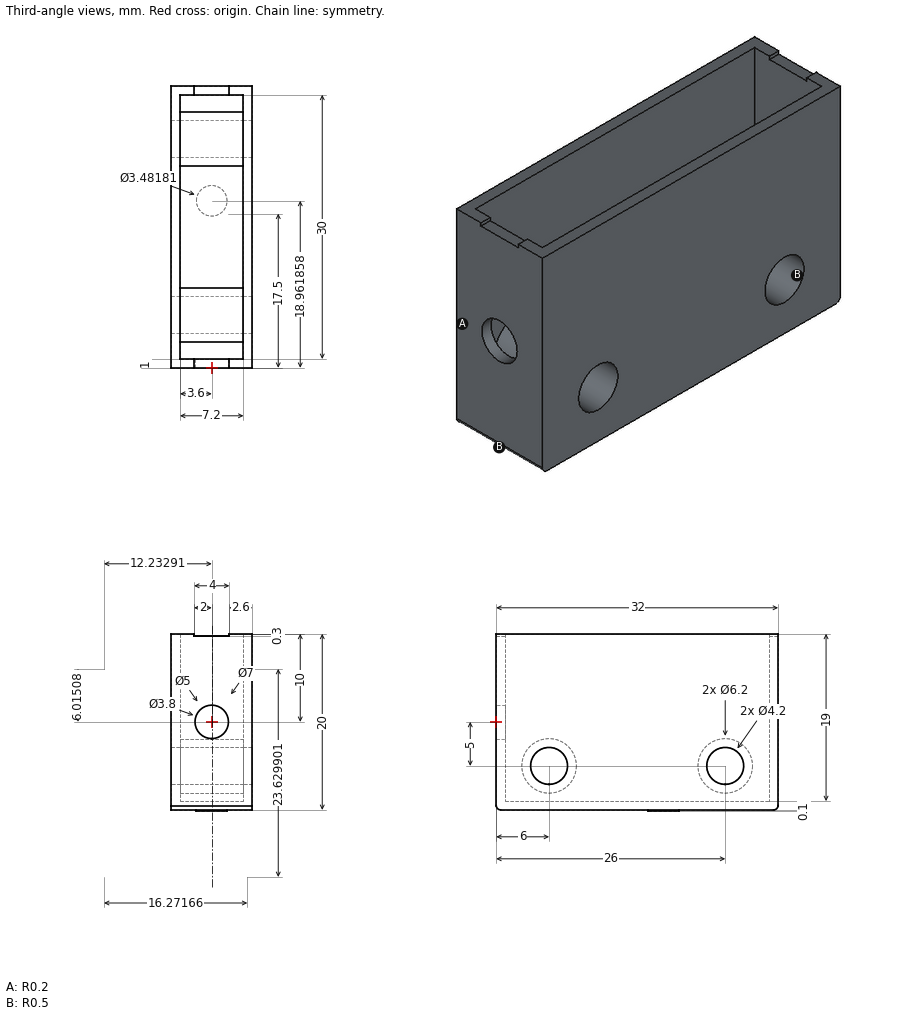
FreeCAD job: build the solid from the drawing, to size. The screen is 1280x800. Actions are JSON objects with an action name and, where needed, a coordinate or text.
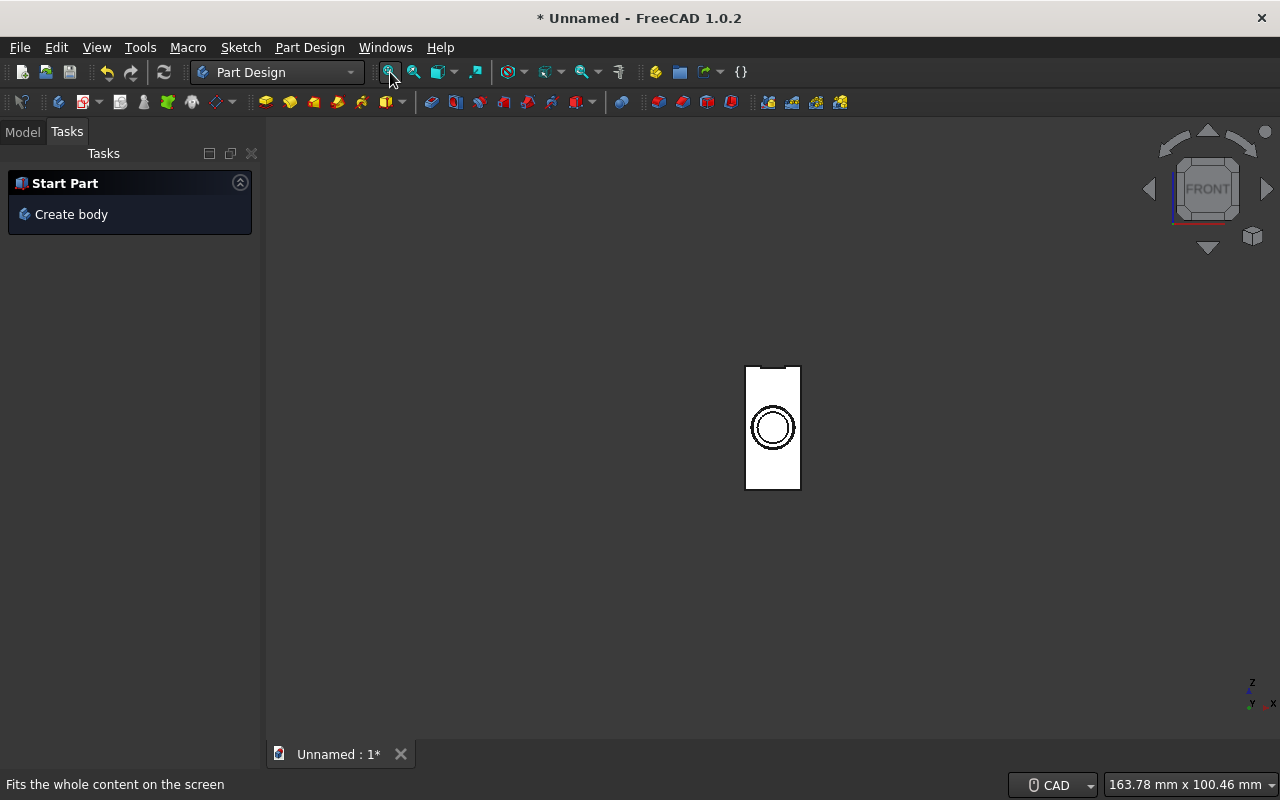
{"action": "key", "text": "3"}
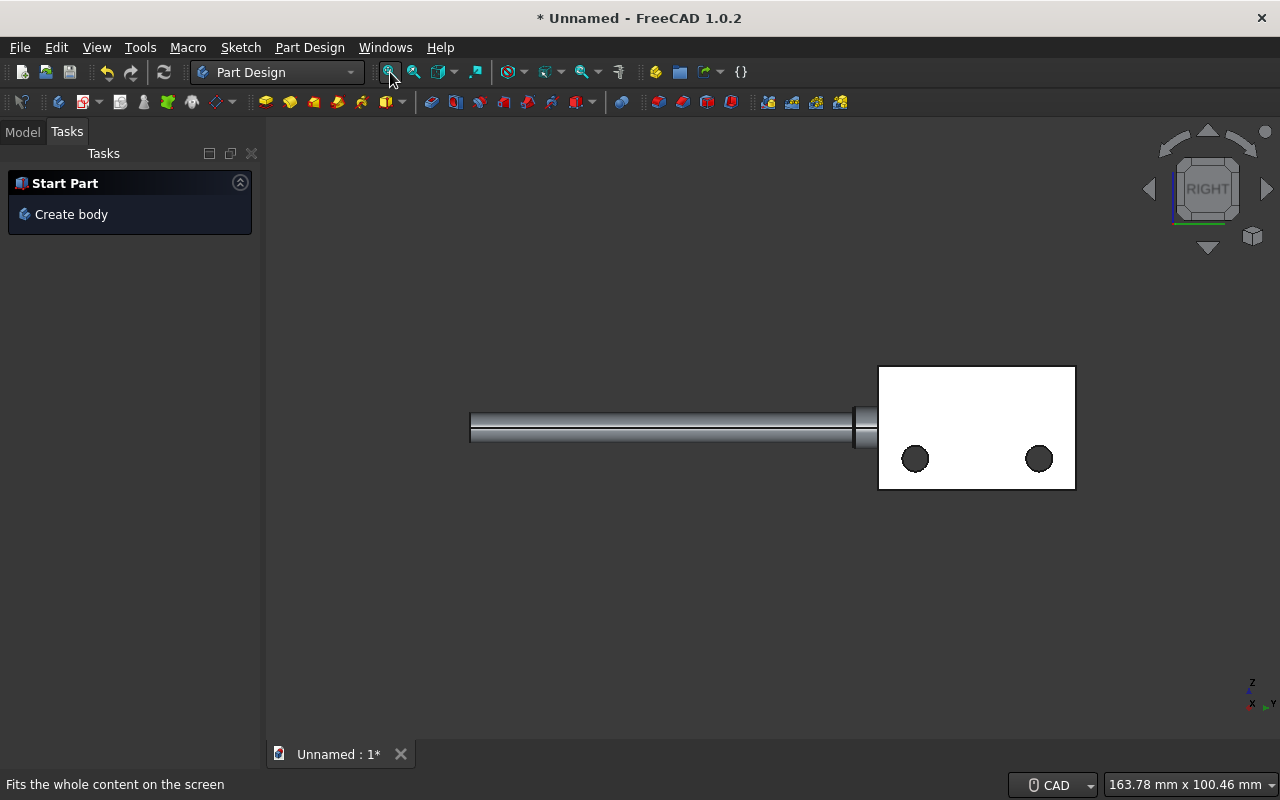
{"action": "key", "text": "5"}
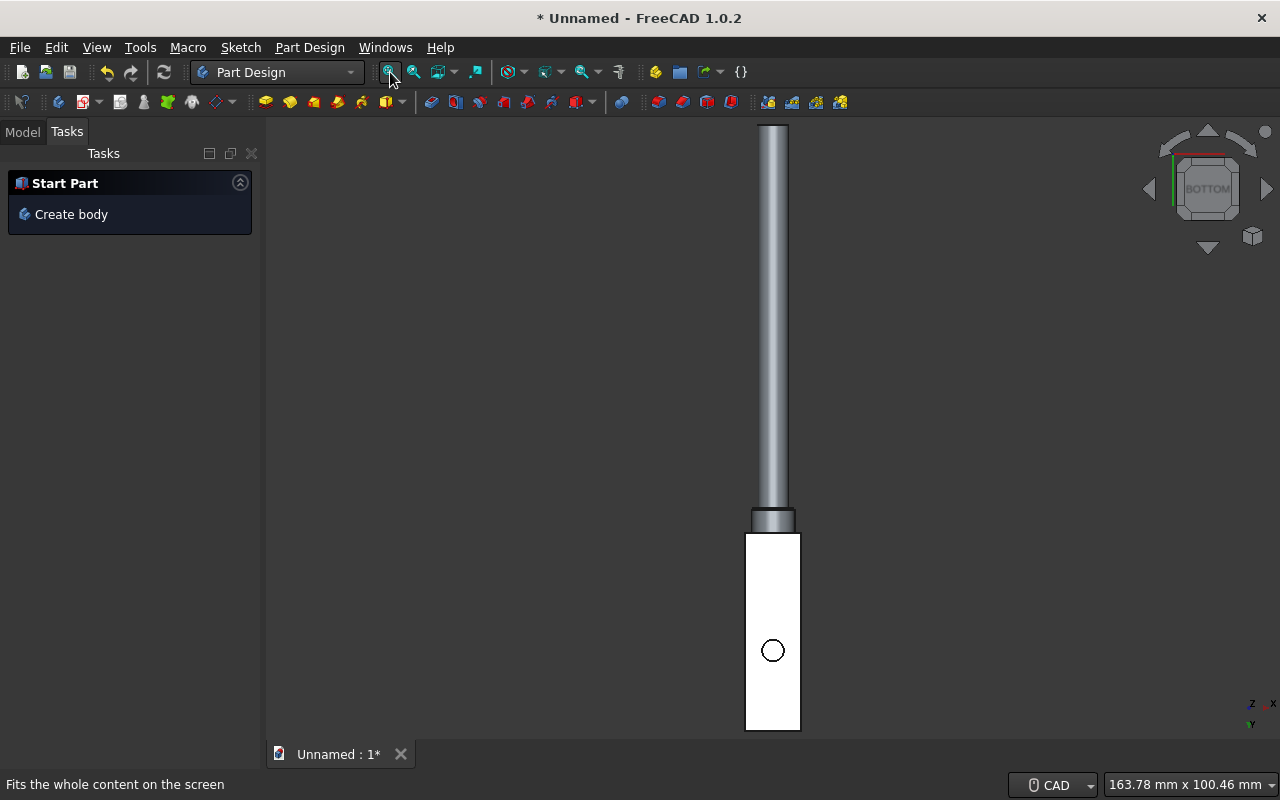
{"action": "left_click", "coordinate": [773, 532]}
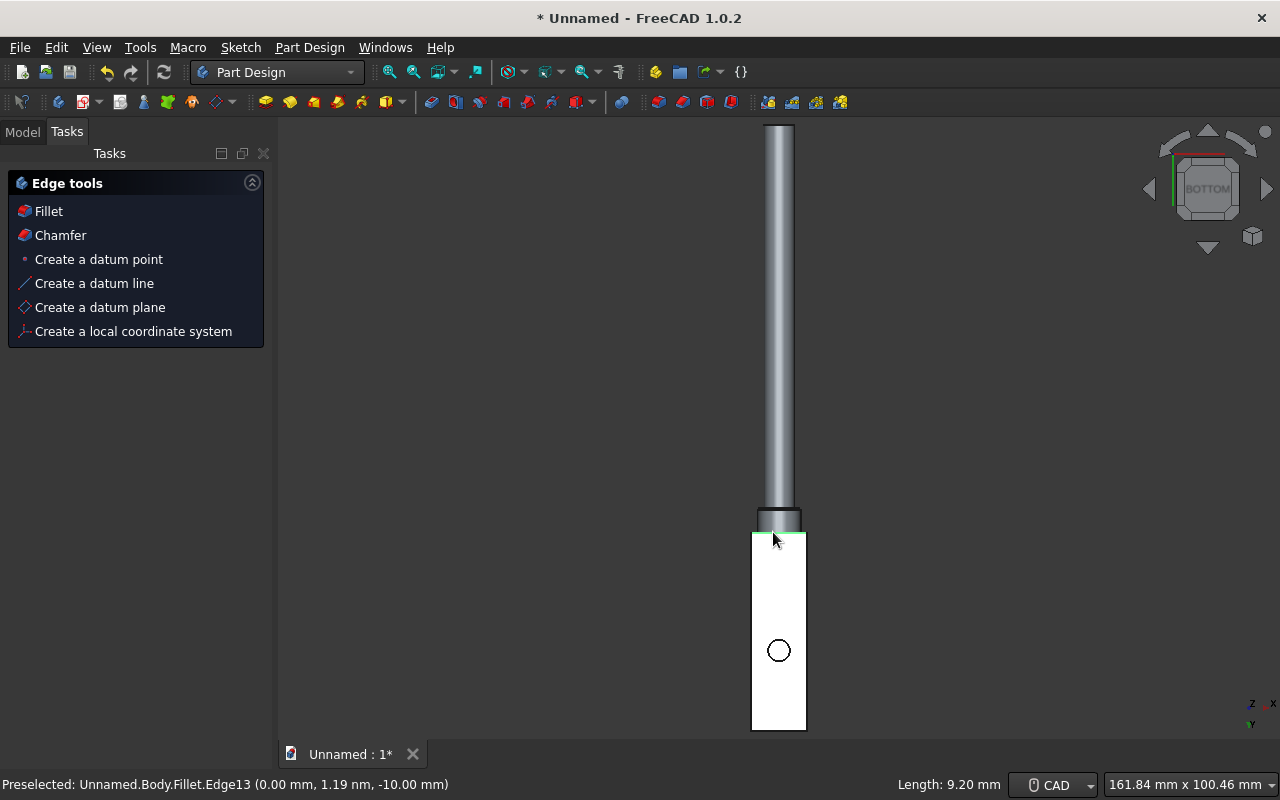
{"action": "key", "text": "4"}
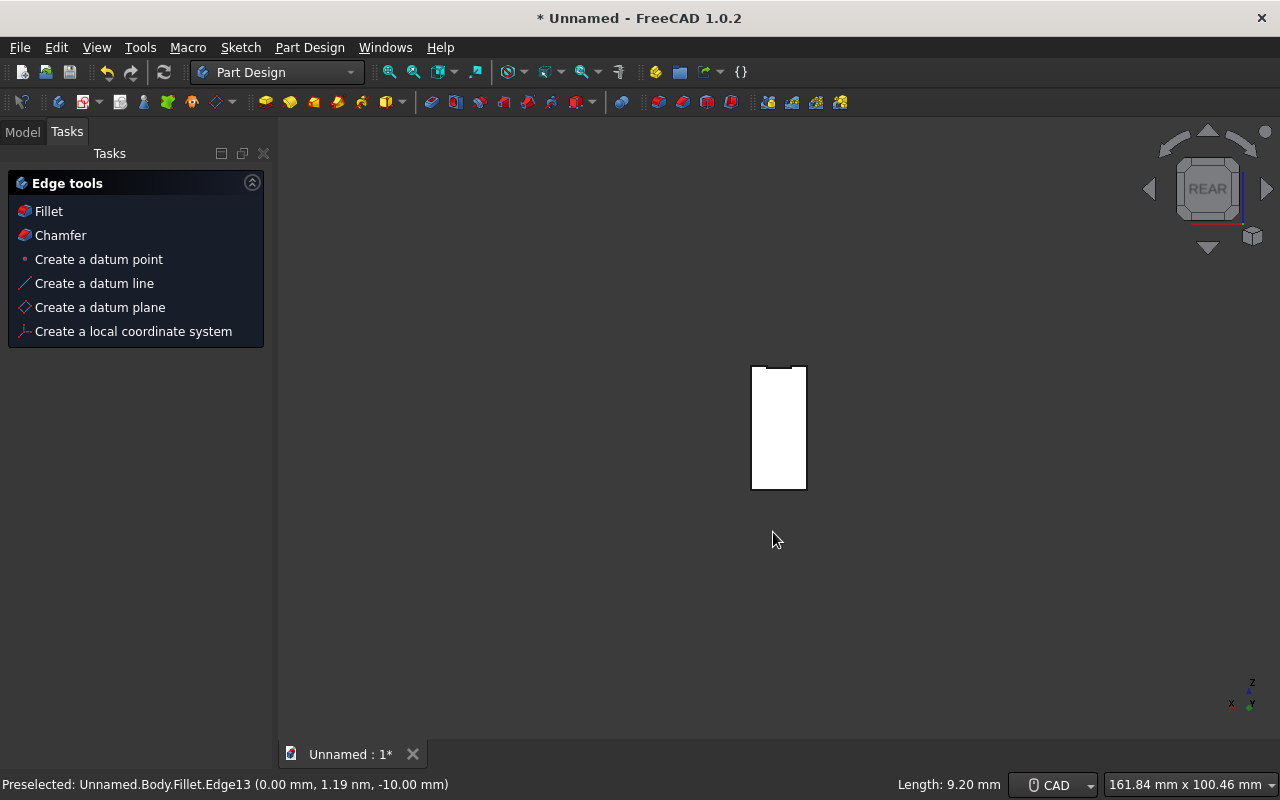
{"action": "left_click", "coordinate": [390, 72]}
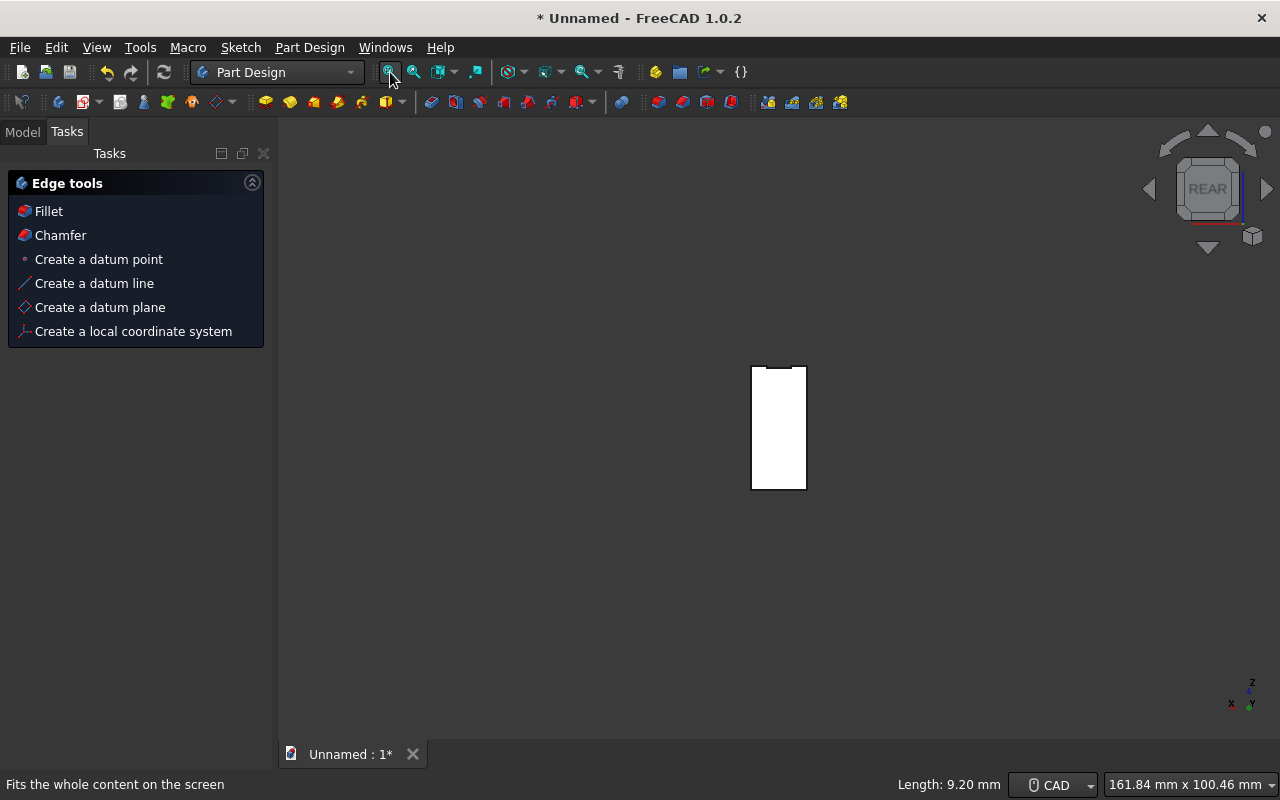
{"action": "left_click", "coordinate": [779, 489], "text": "ctrl"}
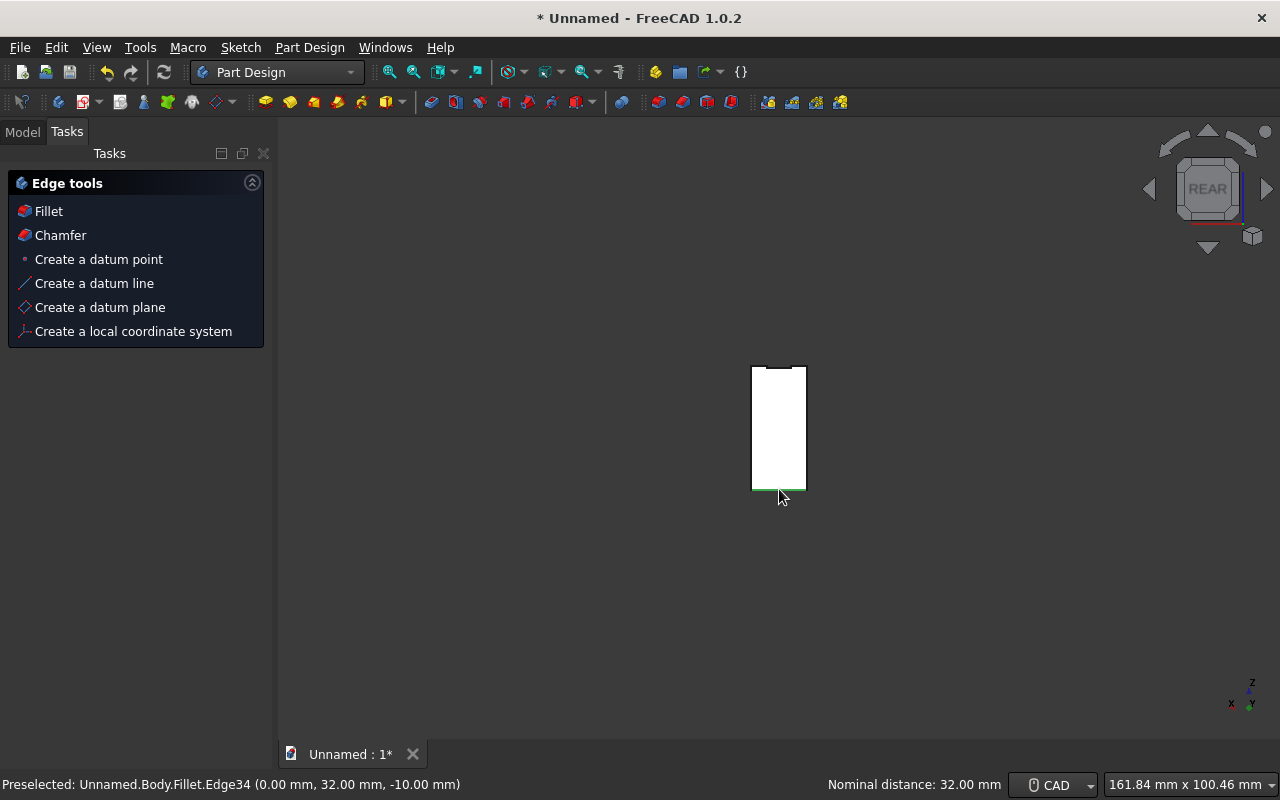
{"action": "left_click", "coordinate": [660, 102]}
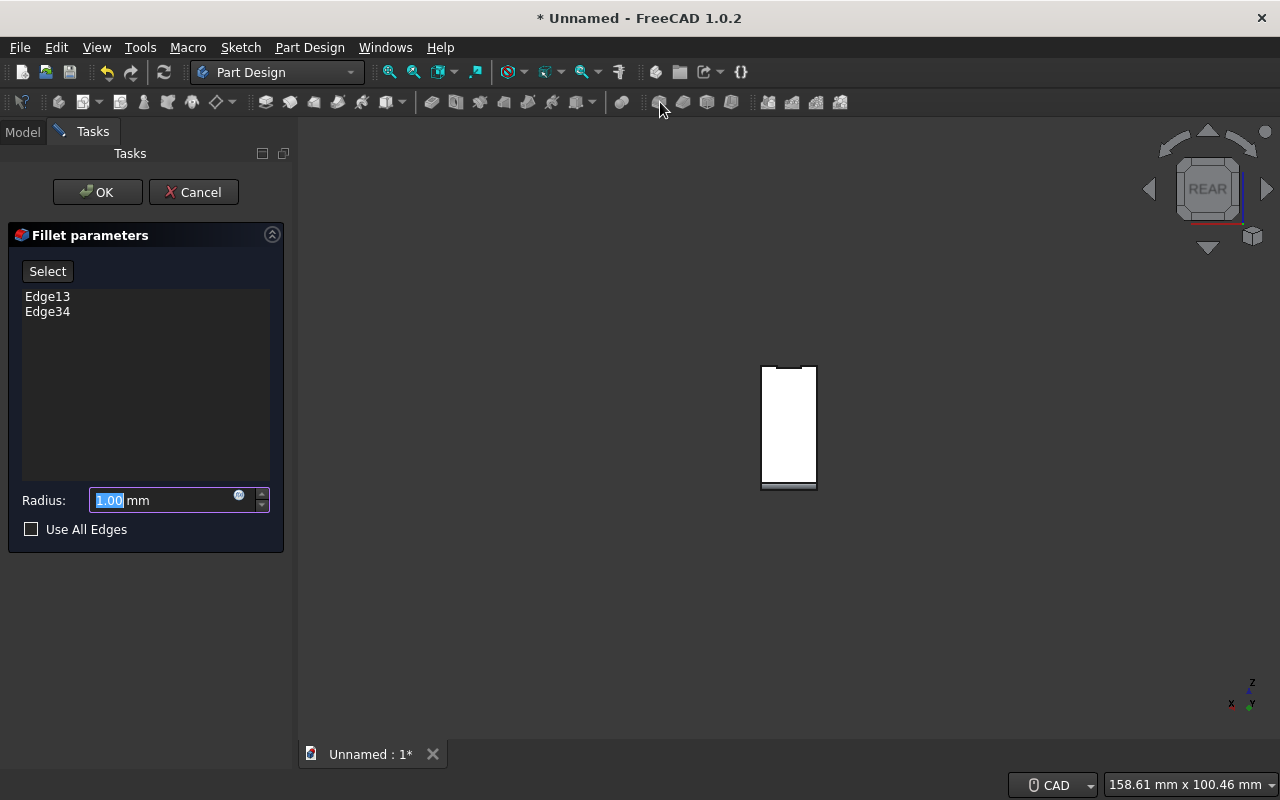
{"action": "type", "text": "0.5"}
{"action": "key", "text": "Tab"}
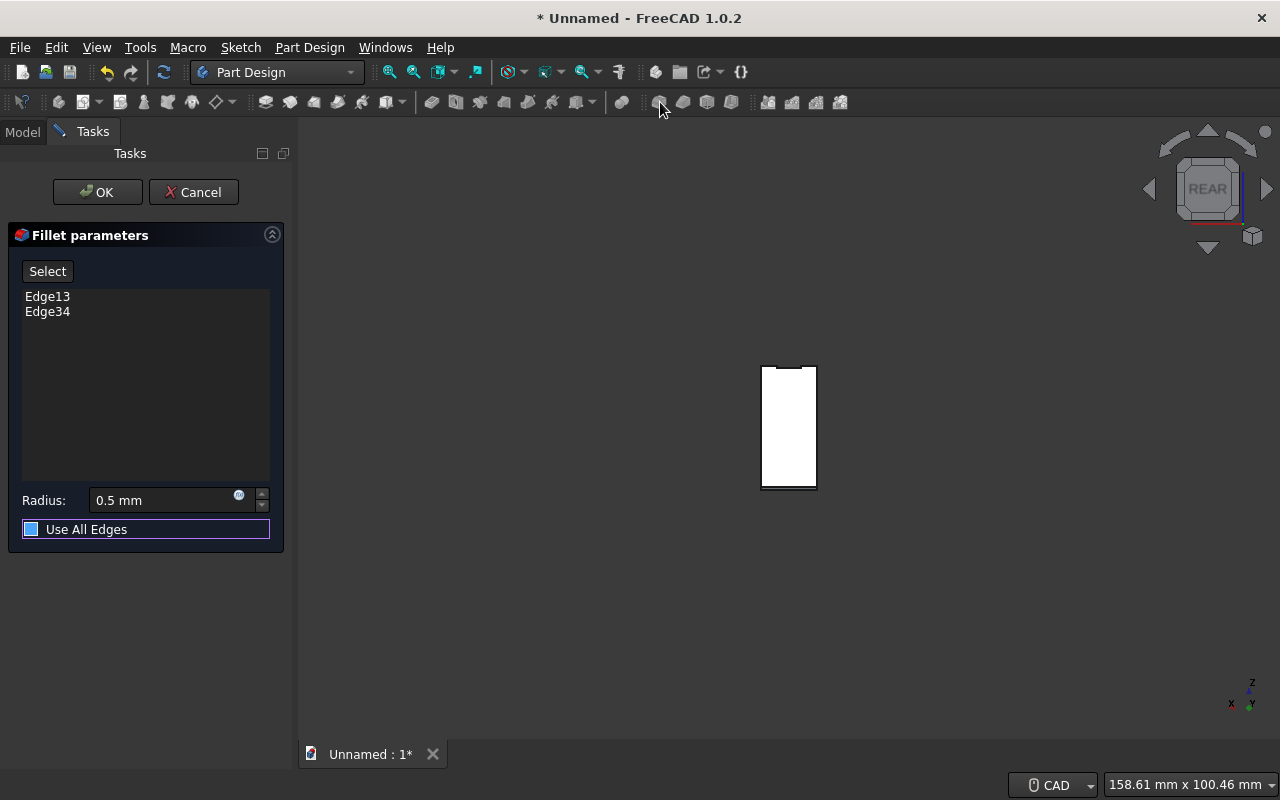
{"action": "left_click", "coordinate": [98, 192]}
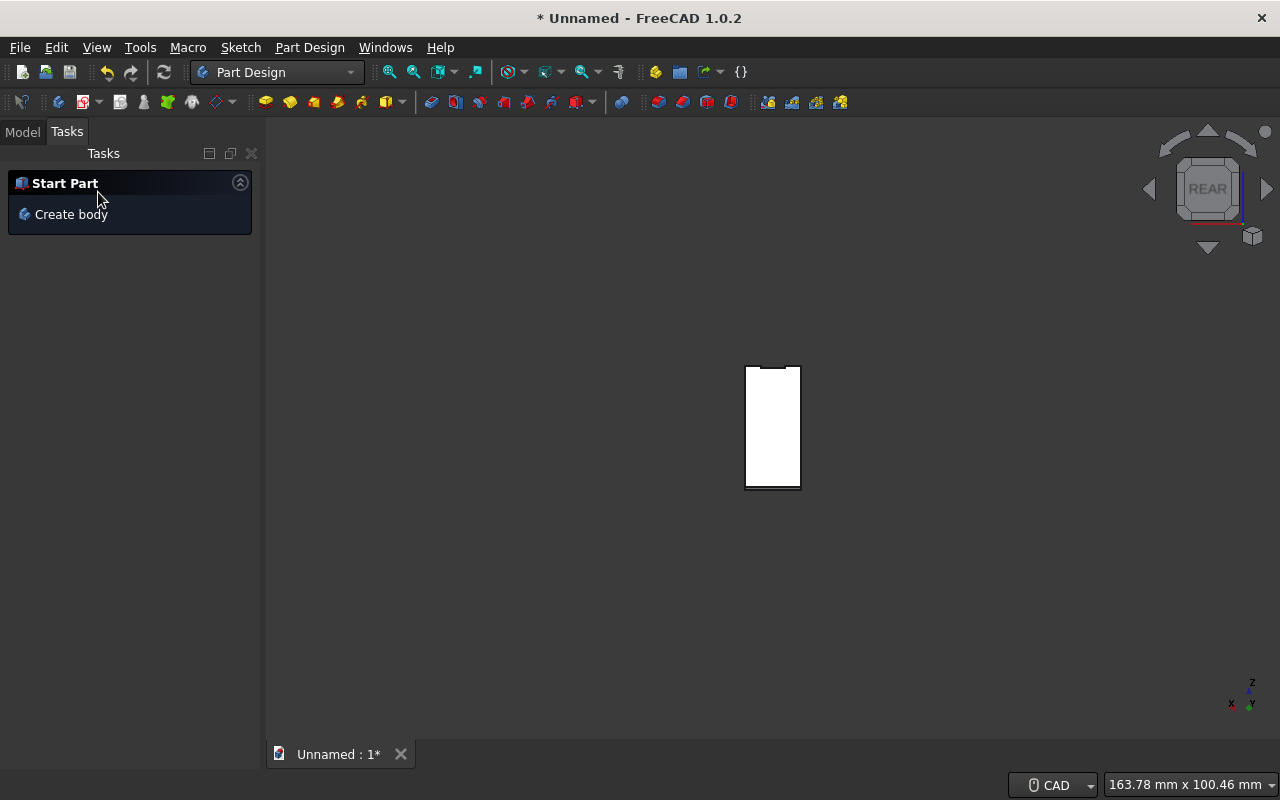
{"action": "left_click", "coordinate": [390, 72]}